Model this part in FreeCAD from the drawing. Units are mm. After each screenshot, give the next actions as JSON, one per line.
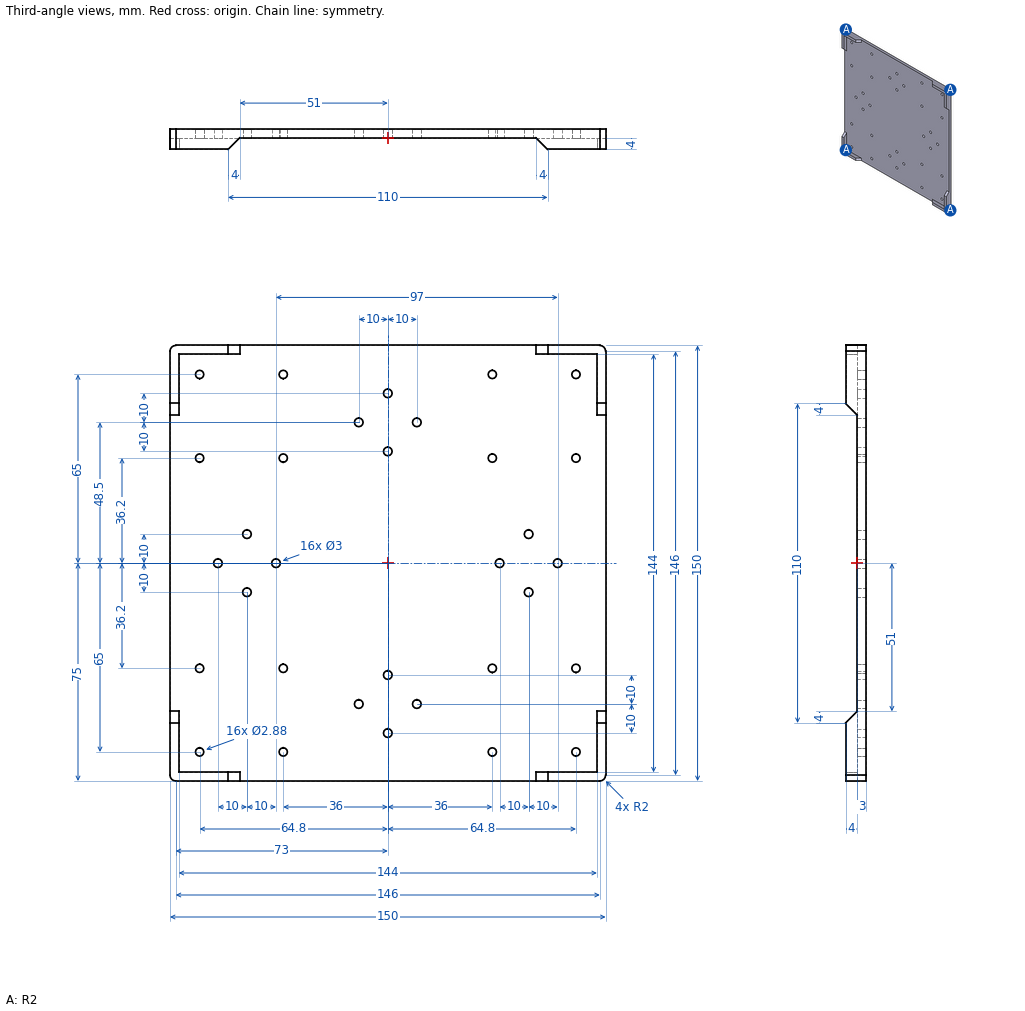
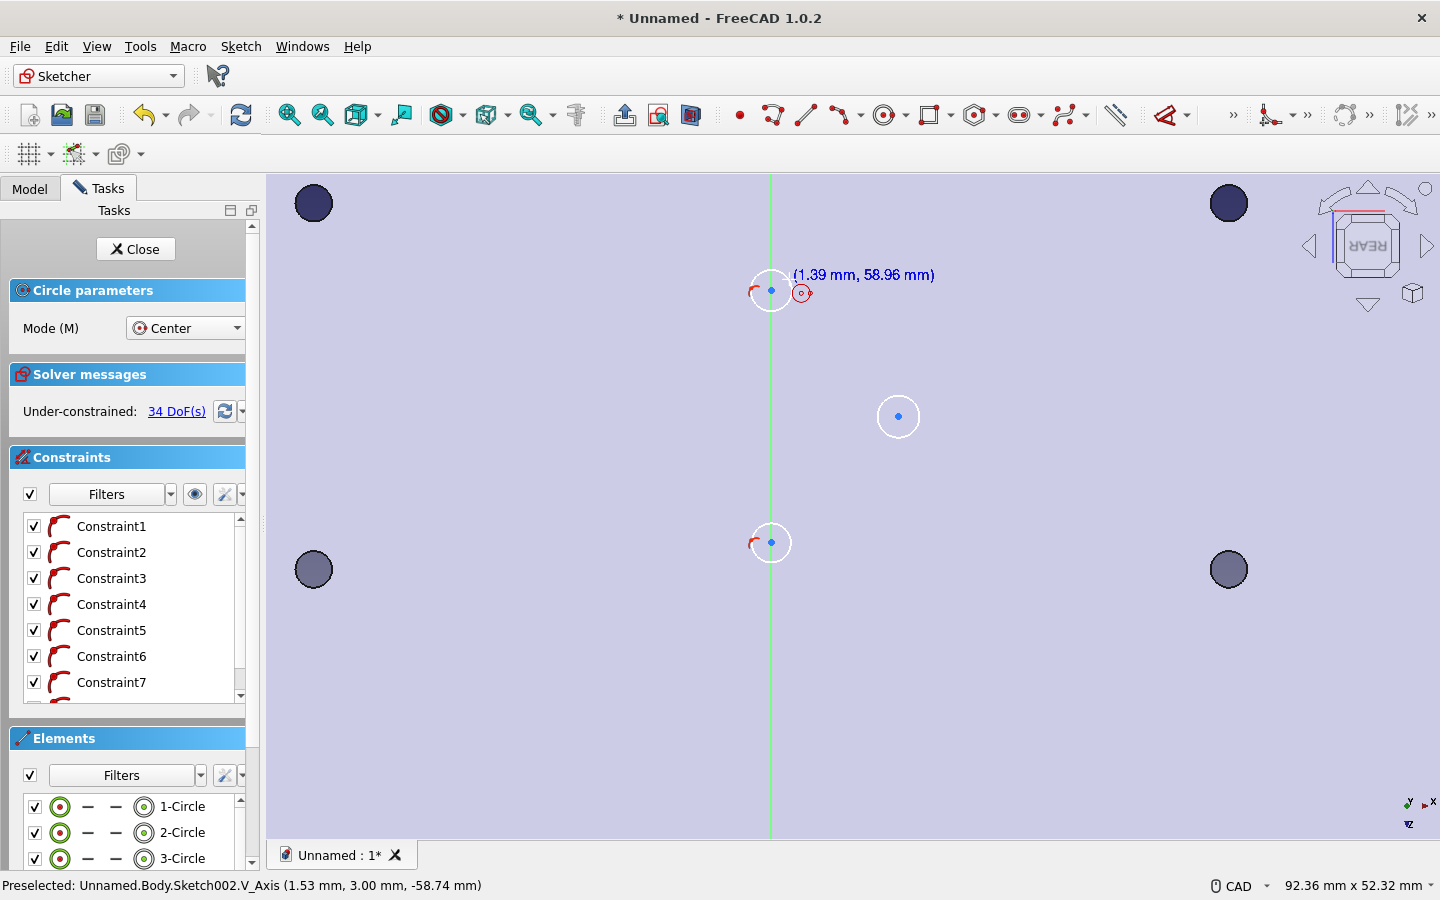
{"action": "scroll", "coordinate": [790, 281], "scroll_direction": "down", "scroll_amount": 6}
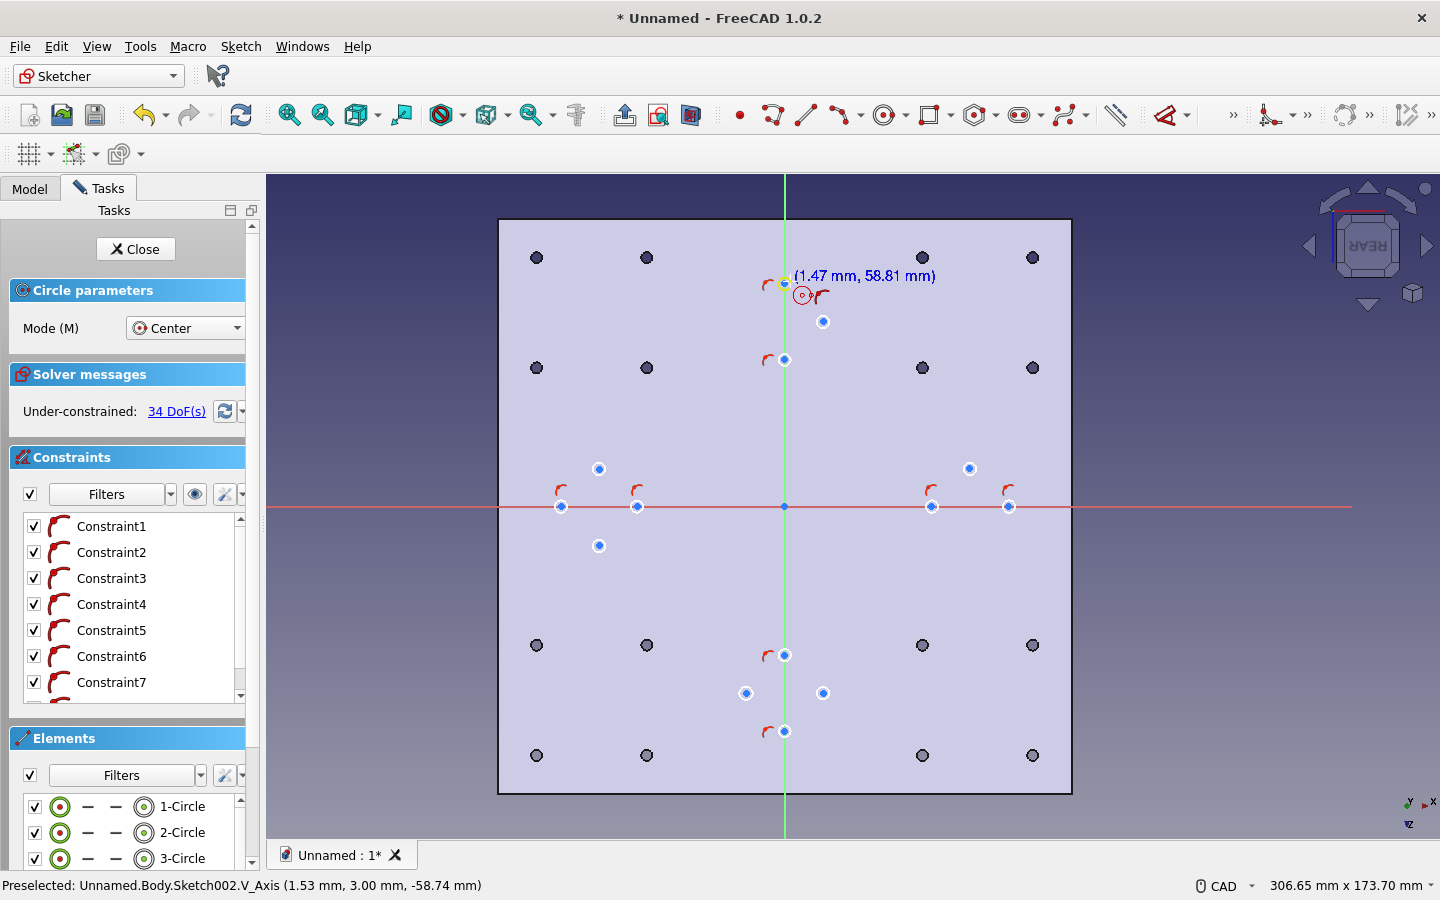
{"action": "left_click", "coordinate": [746, 321]}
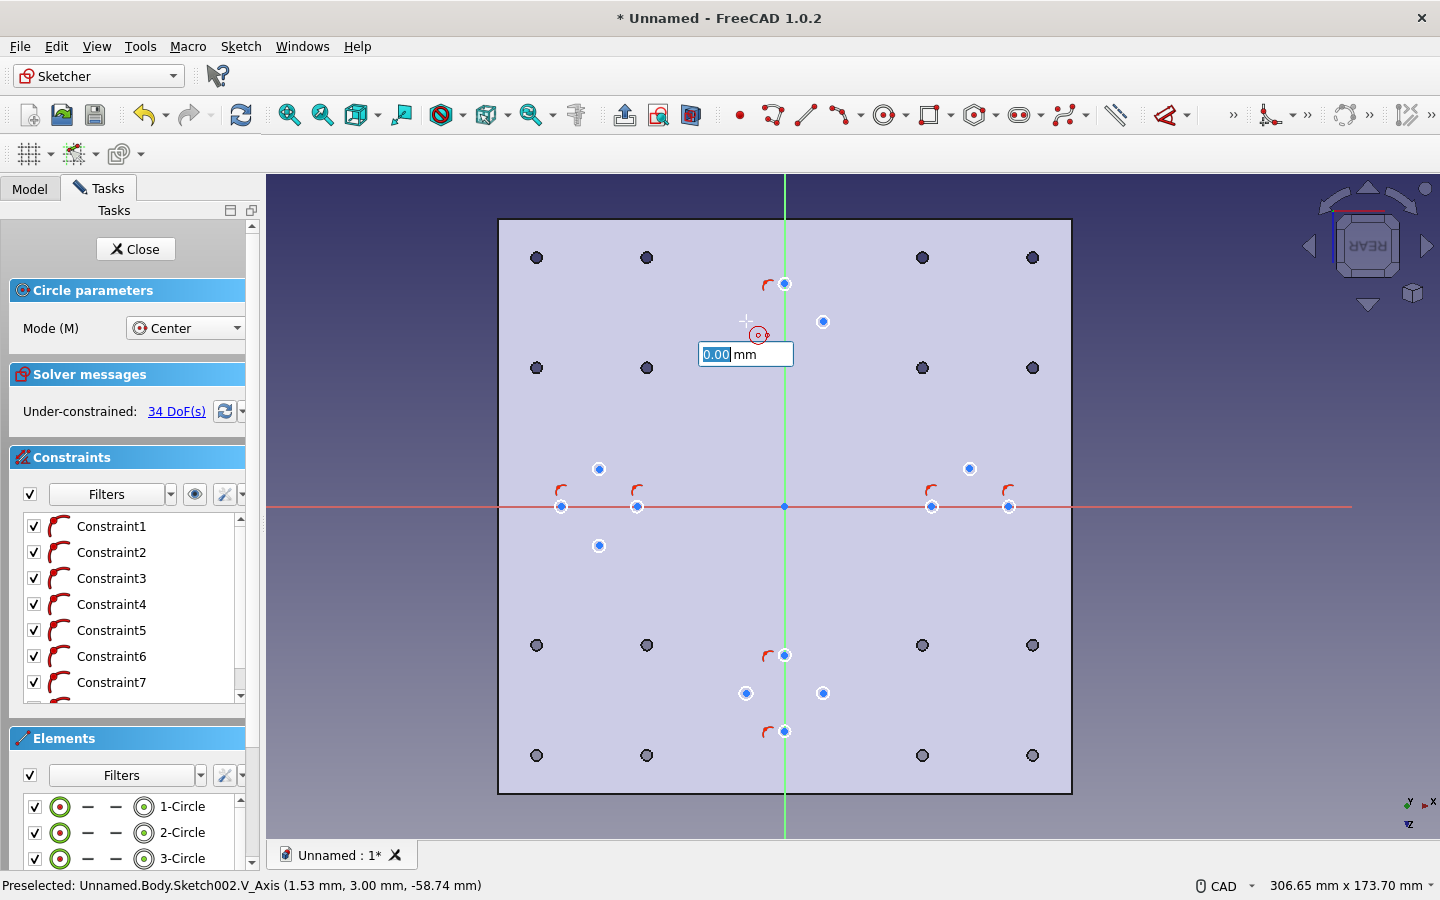
{"action": "scroll", "coordinate": [750, 317], "scroll_direction": "up", "scroll_amount": 6}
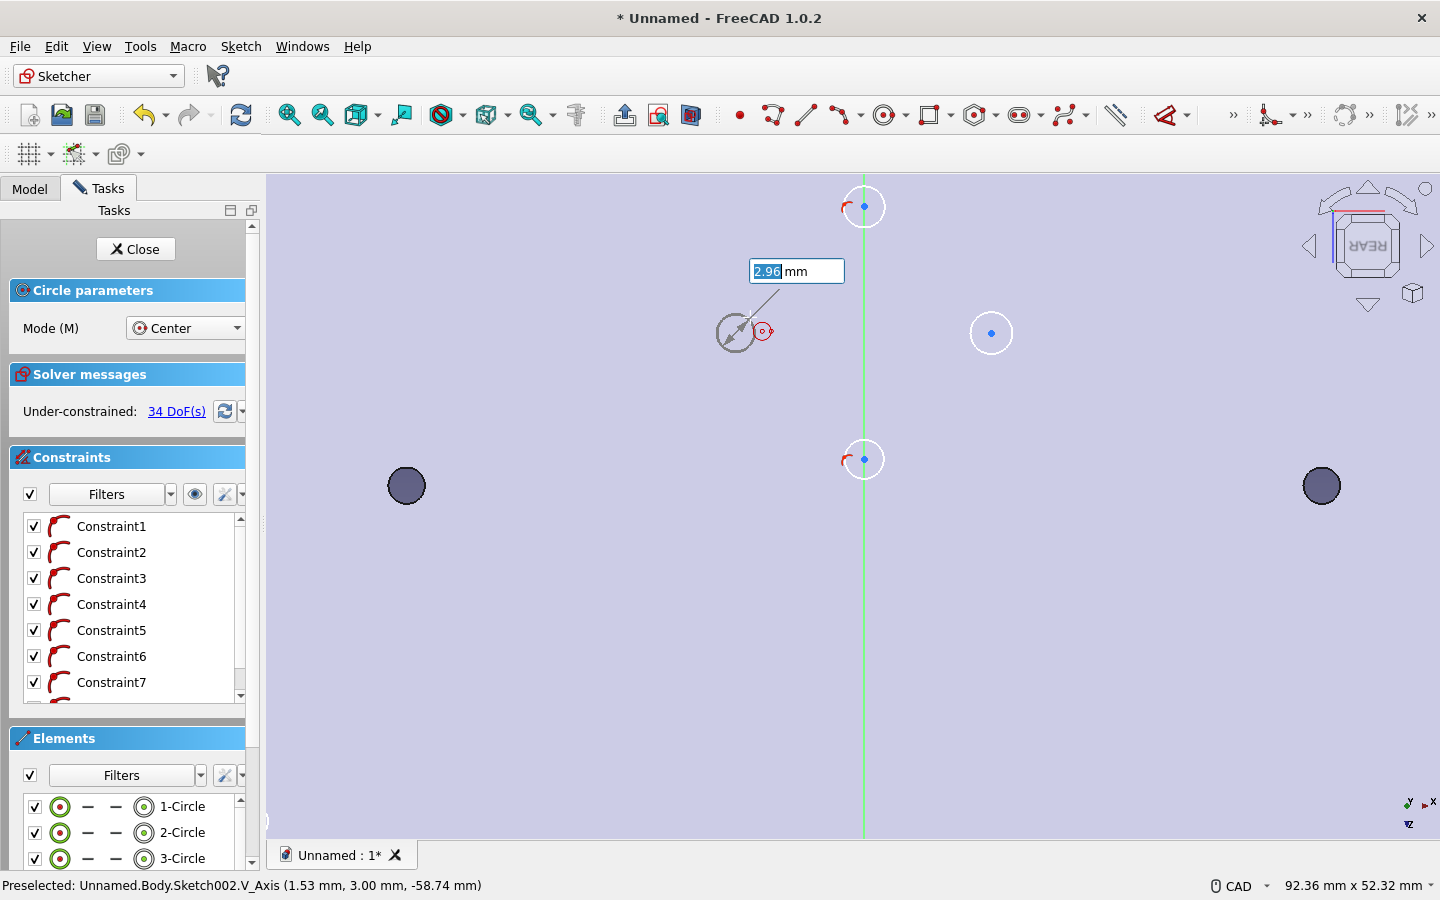
{"action": "left_click", "coordinate": [751, 316]}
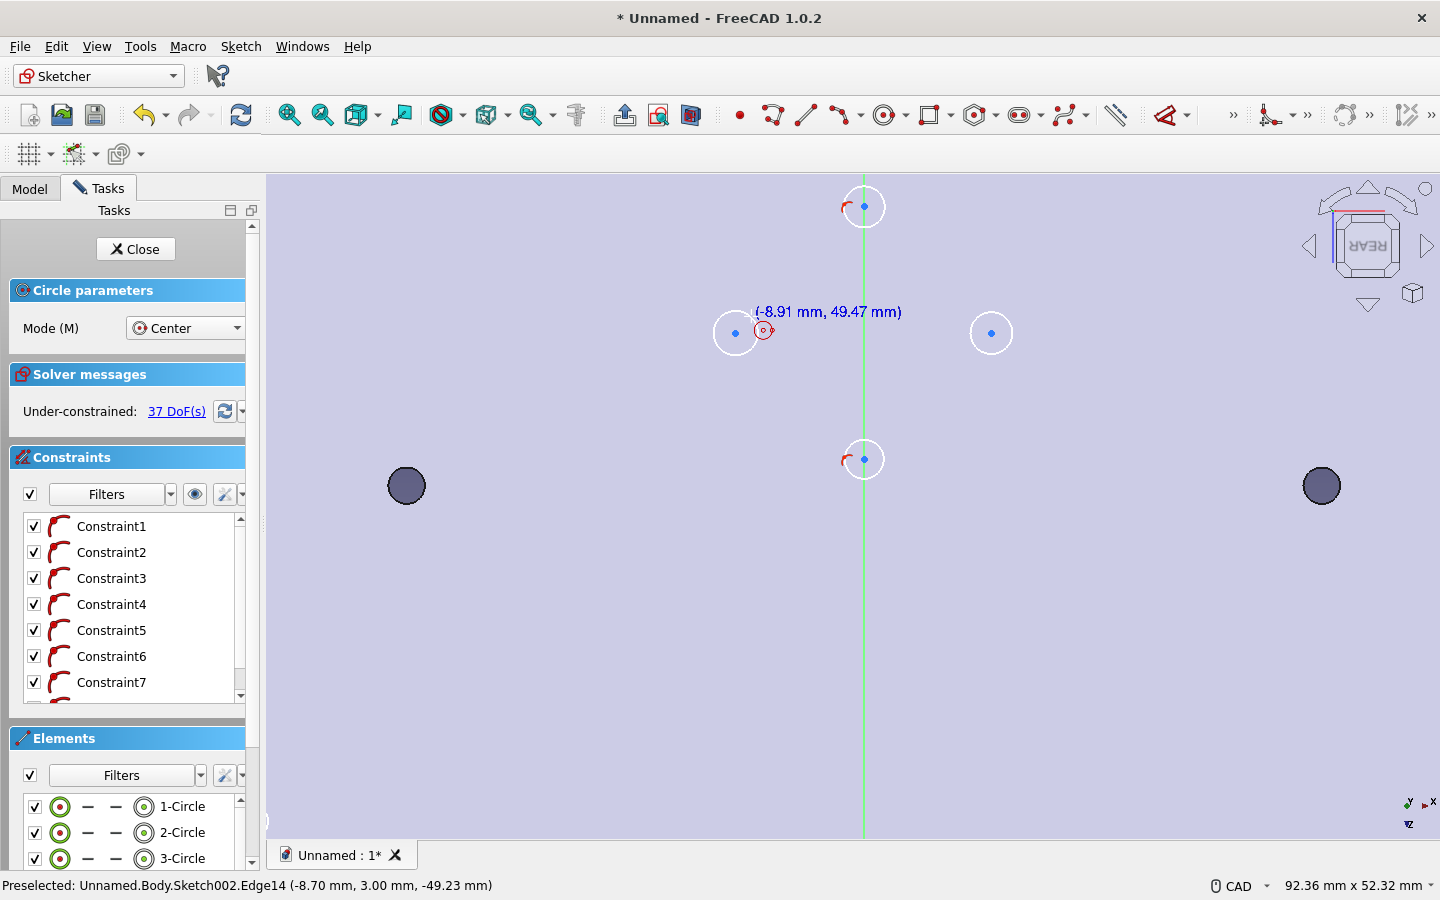
{"action": "scroll", "coordinate": [750, 317], "scroll_direction": "down", "scroll_amount": 6}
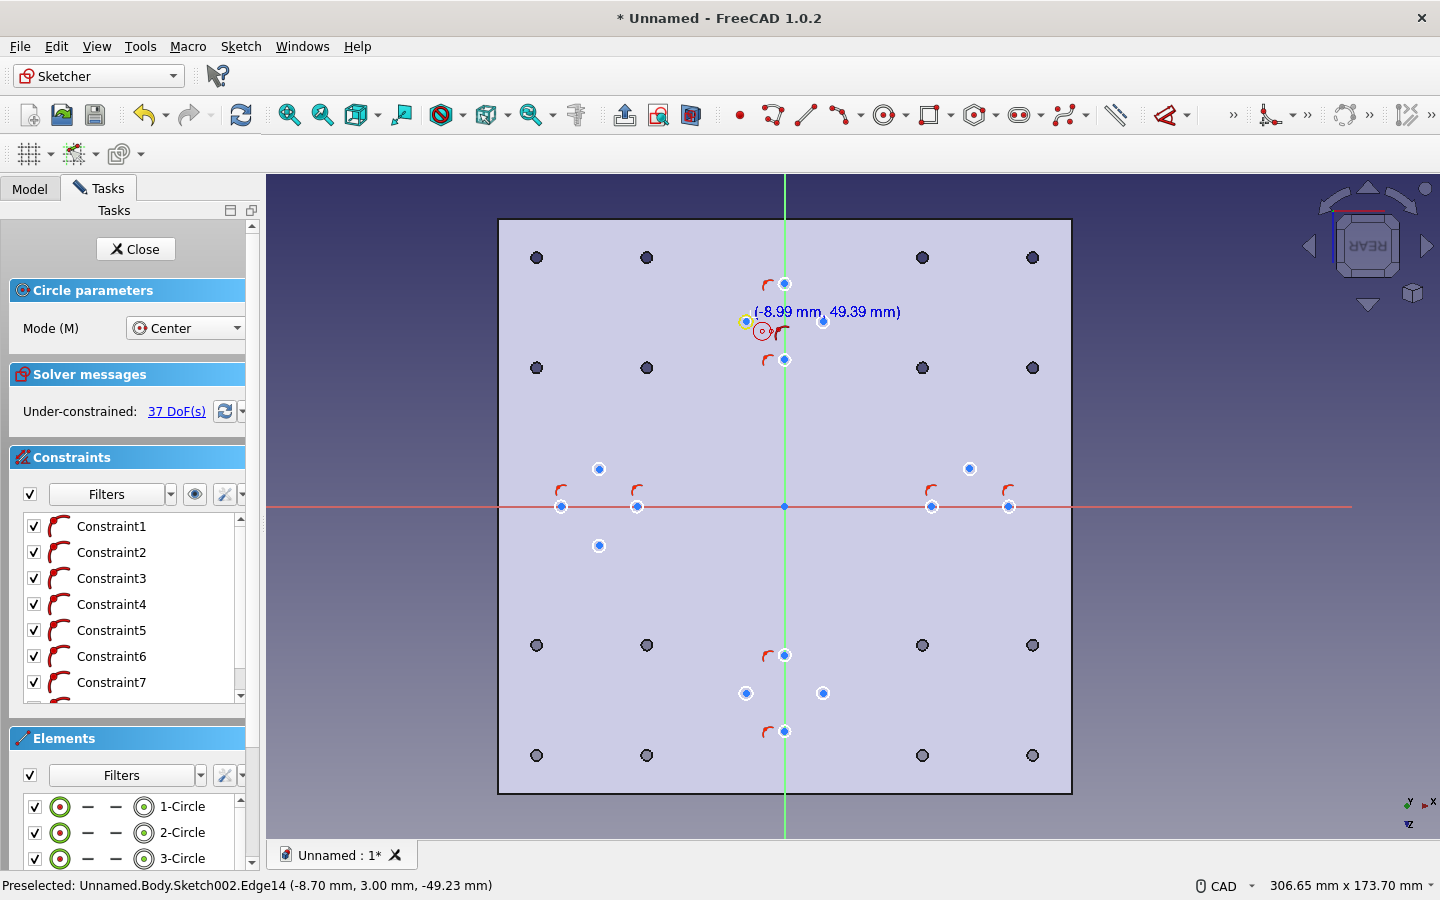
{"action": "scroll", "coordinate": [970, 545], "scroll_direction": "up", "scroll_amount": 7}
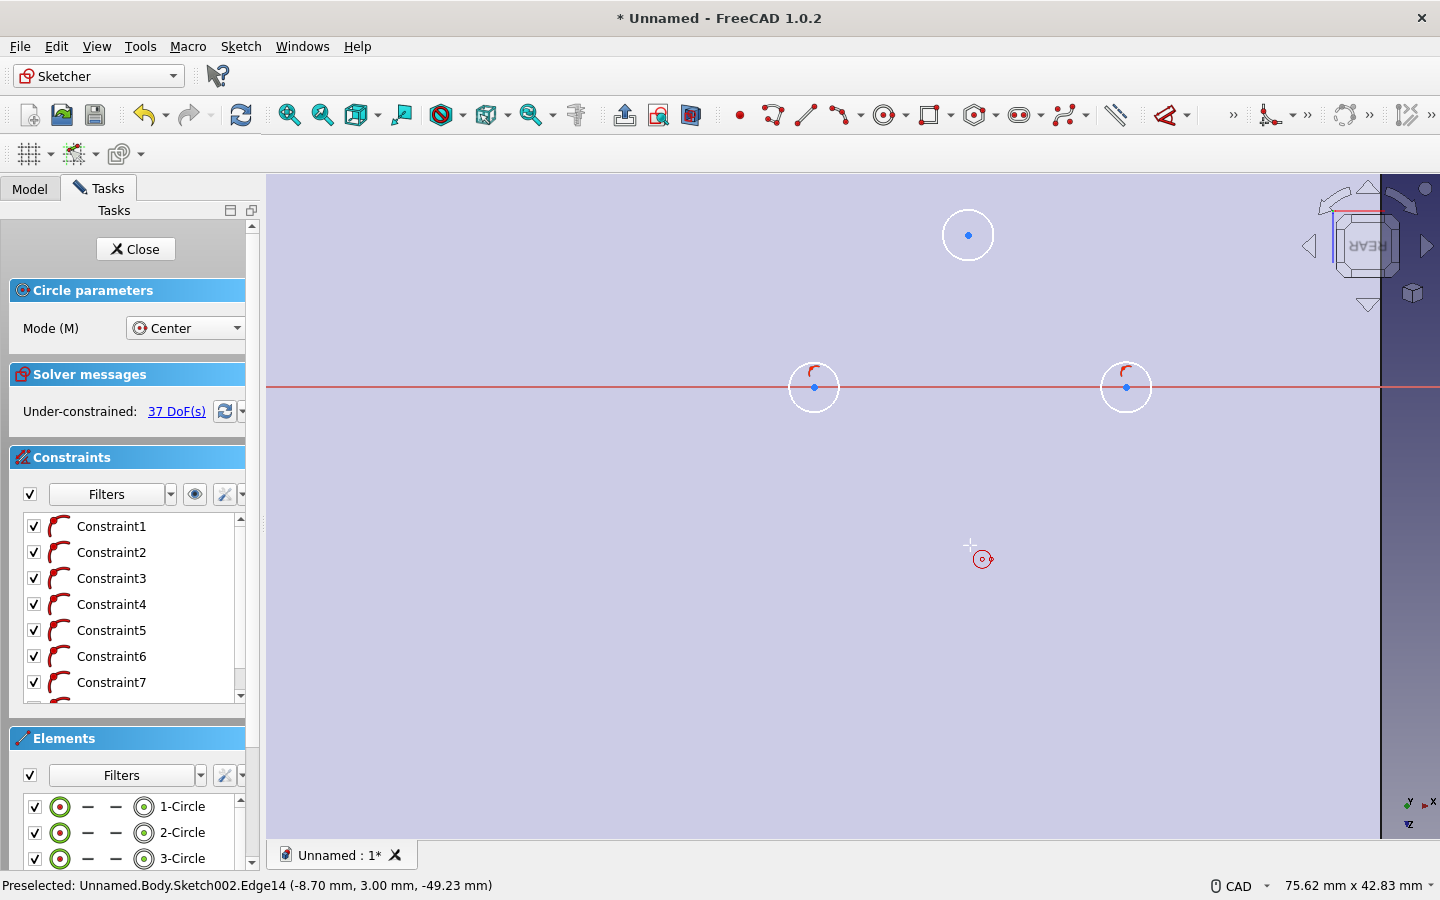
{"action": "scroll", "coordinate": [970, 545], "scroll_direction": "down", "scroll_amount": 7}